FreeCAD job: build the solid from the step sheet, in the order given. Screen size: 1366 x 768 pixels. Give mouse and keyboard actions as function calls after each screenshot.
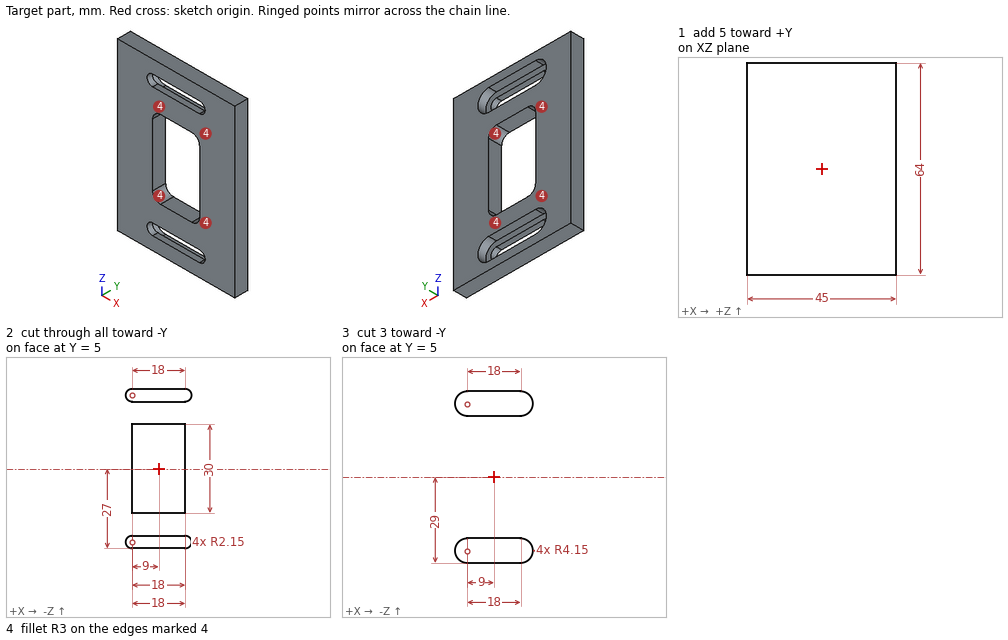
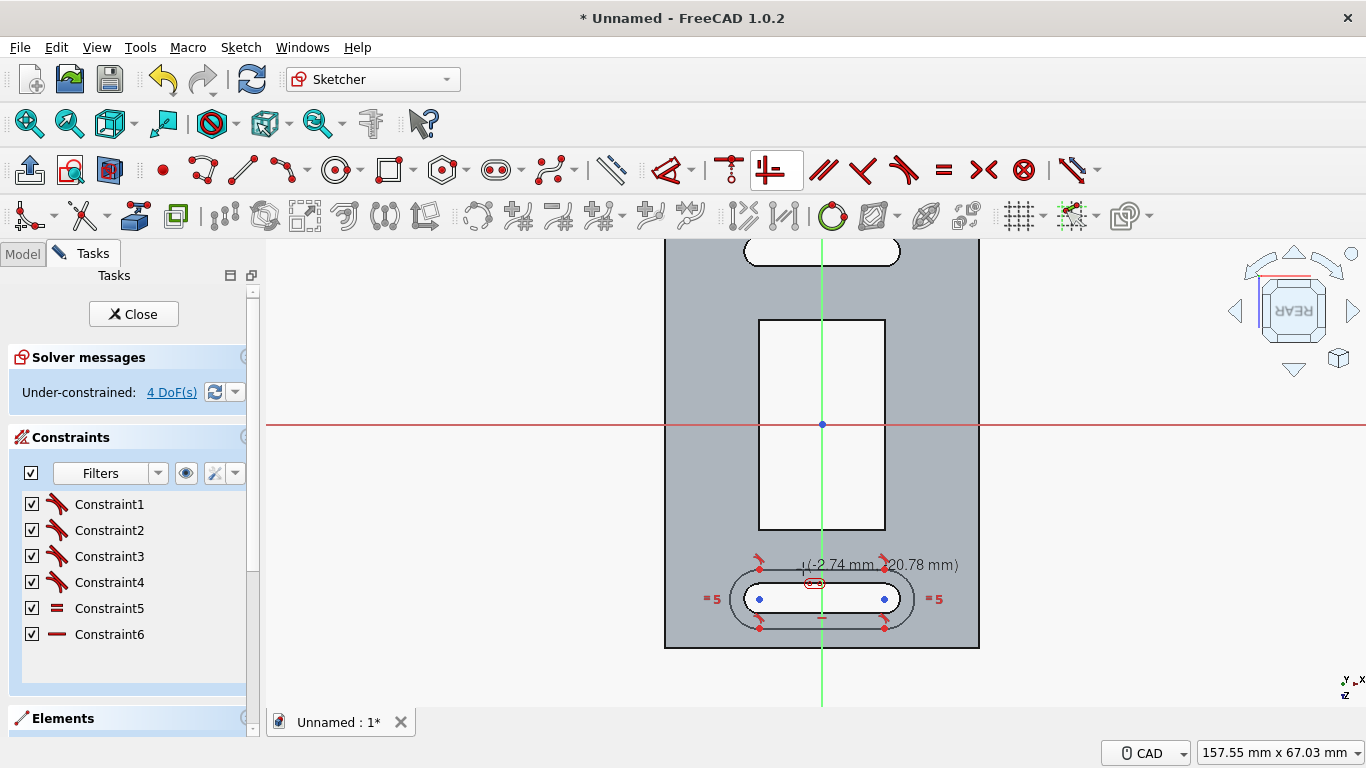
scroll(596, 571, down, 2)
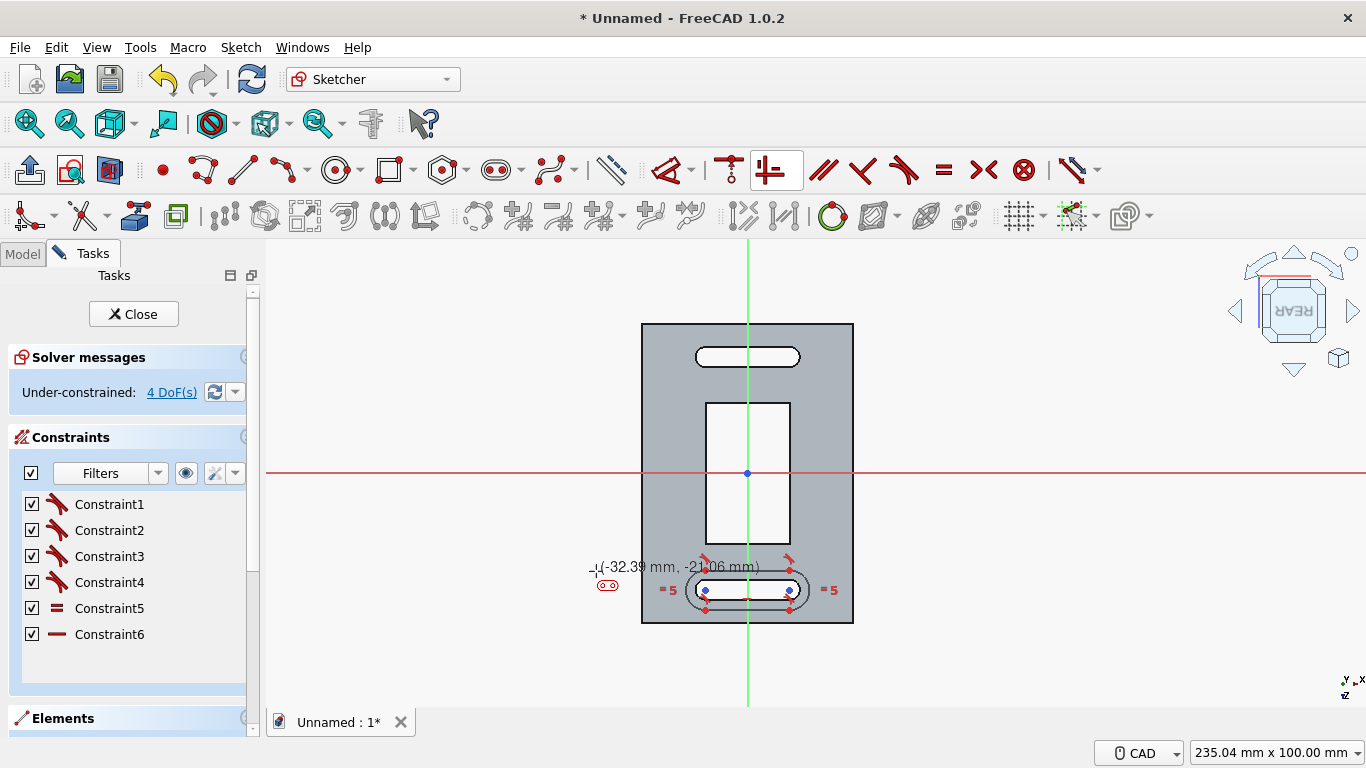
click(706, 357)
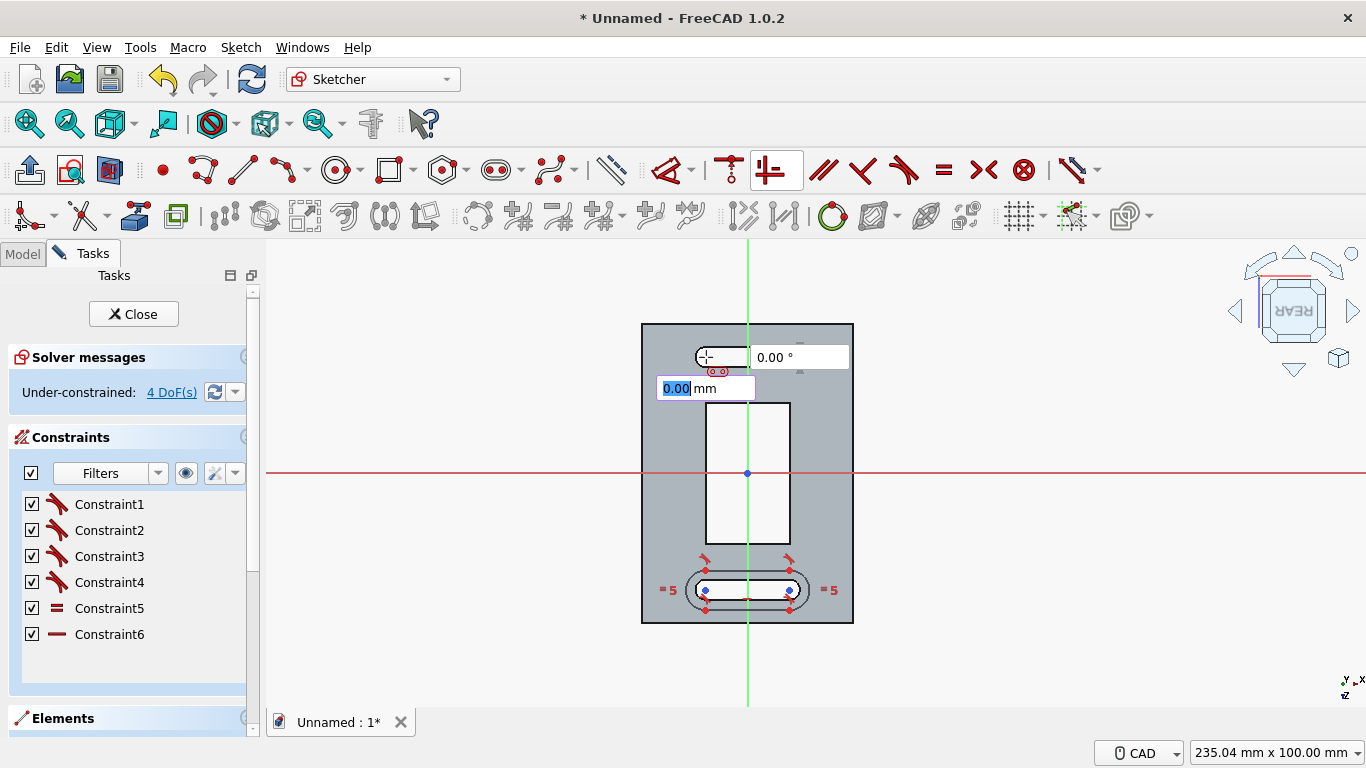
click(790, 357)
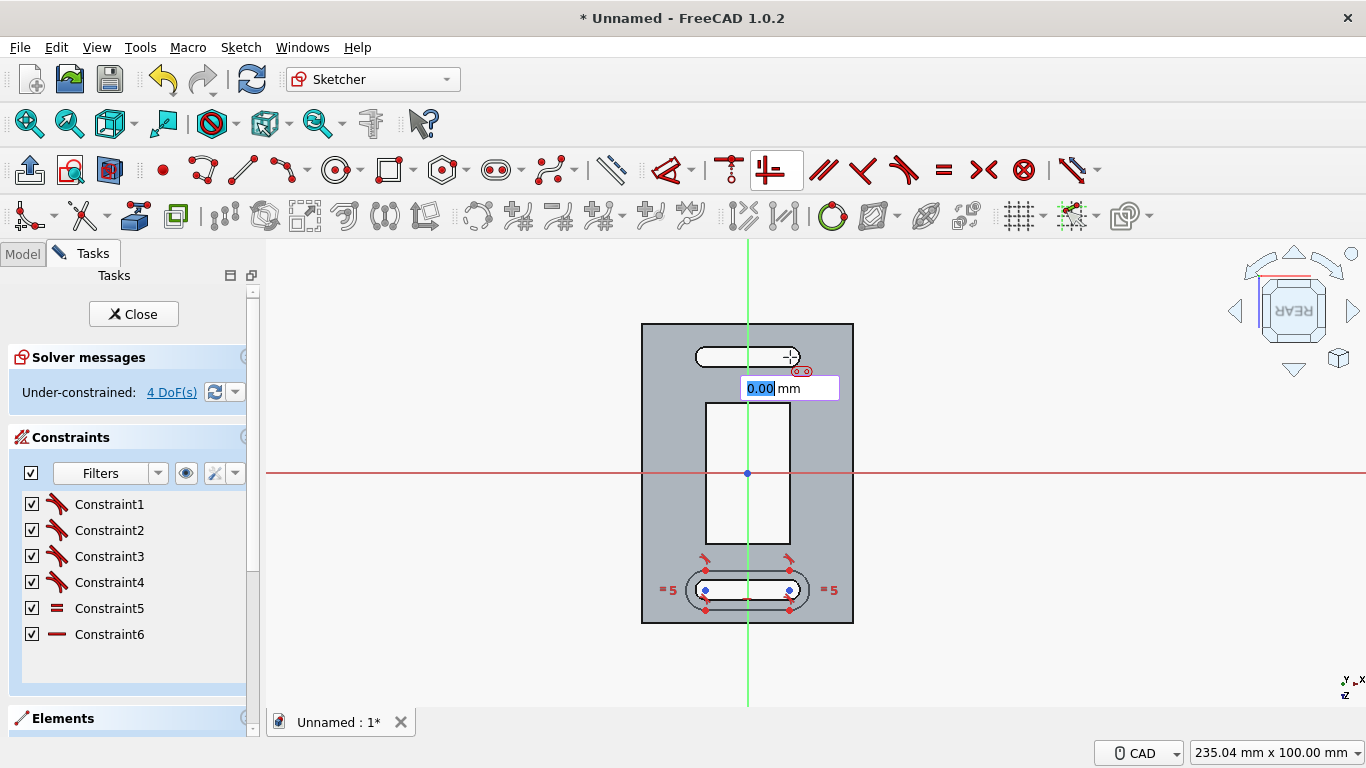
scroll(760, 376, up, 2)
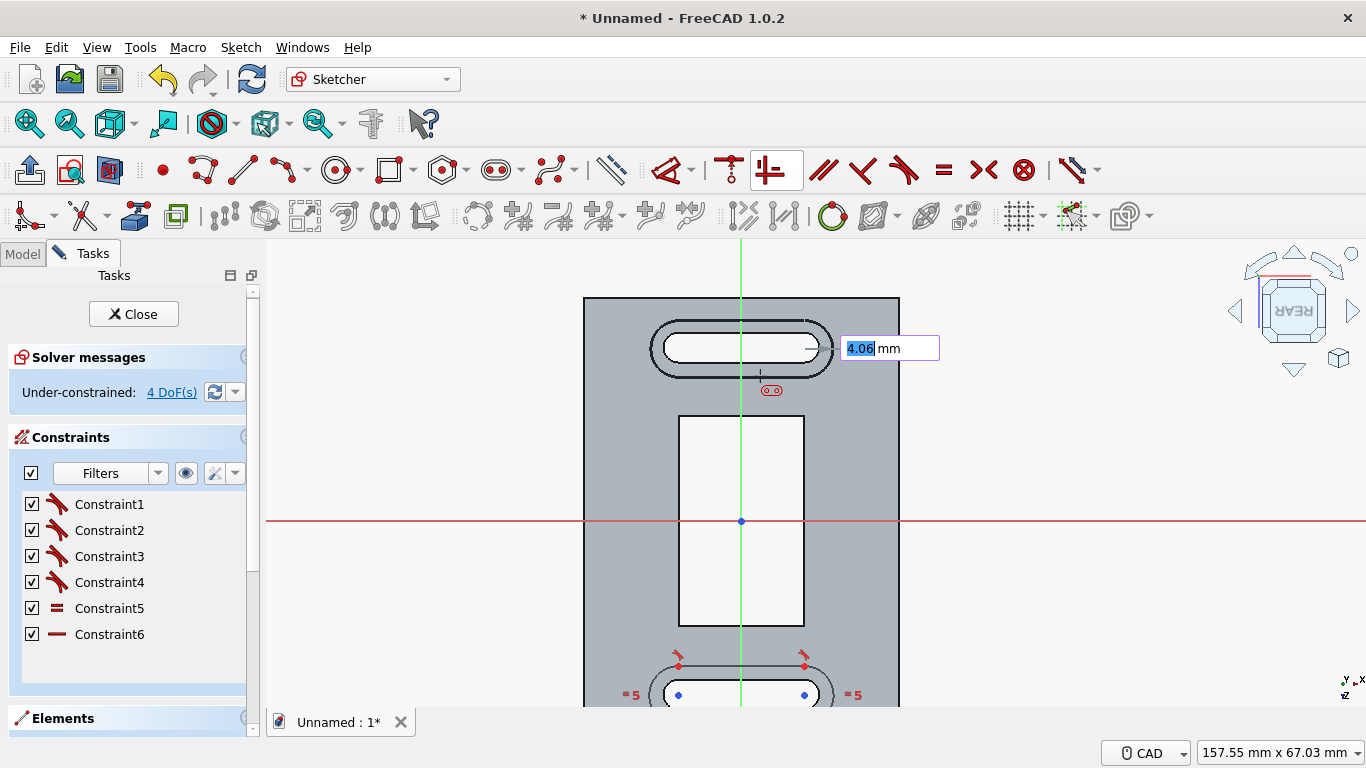
click(760, 377)
key(Escape)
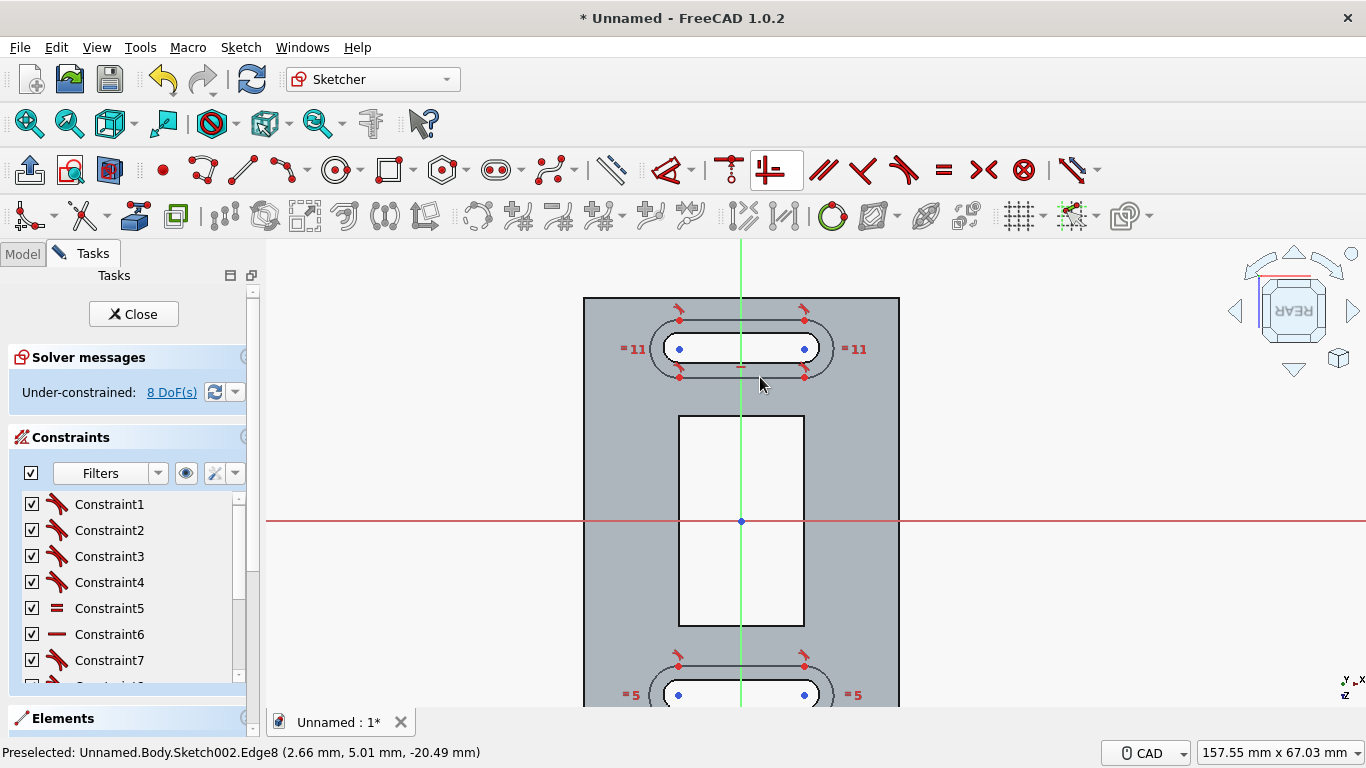
click(655, 678)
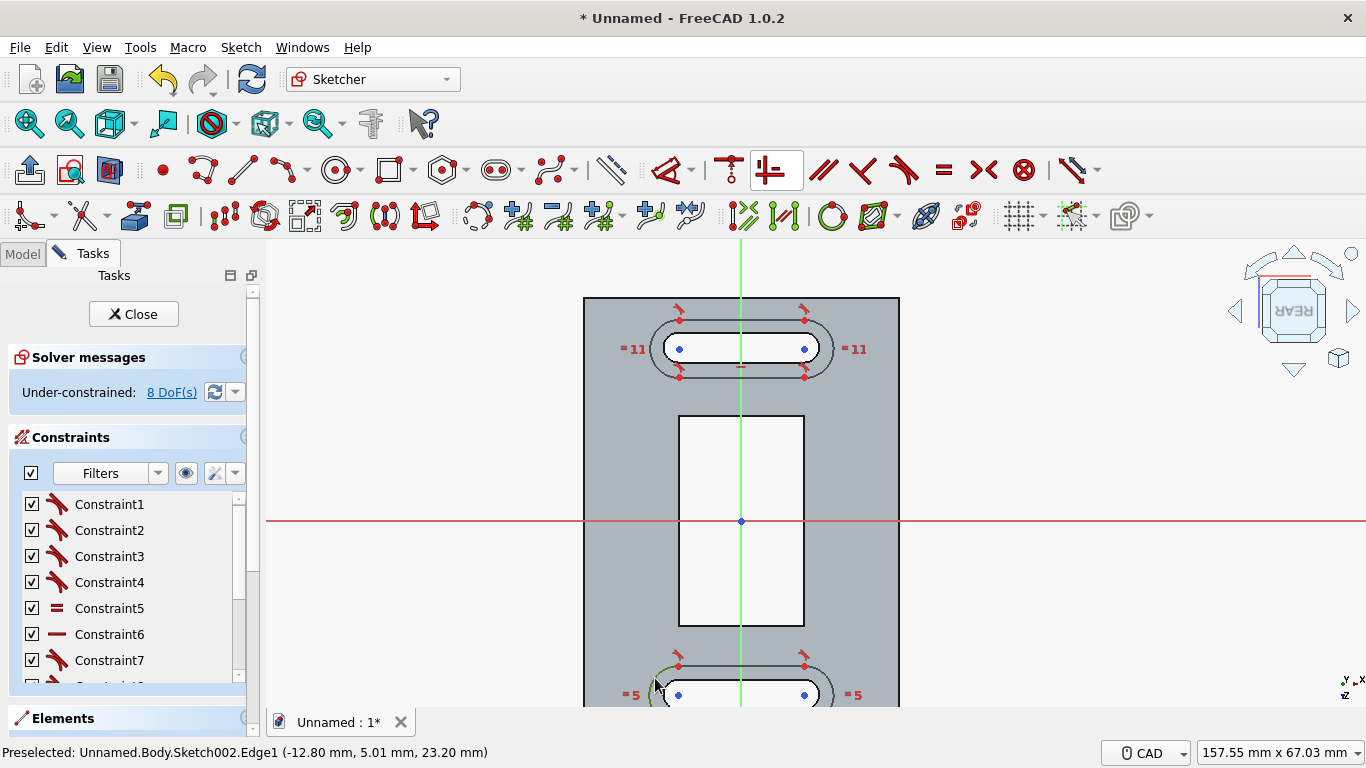
click(656, 332)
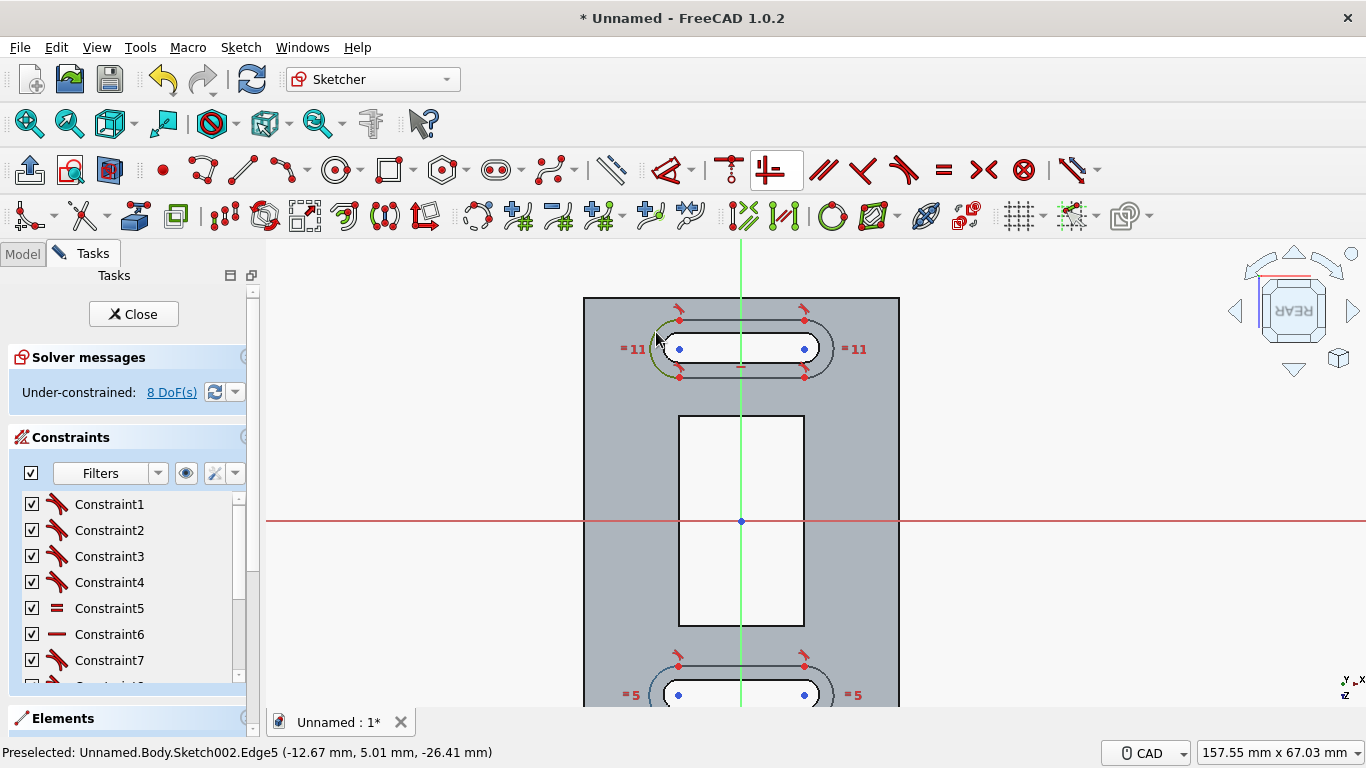
click(944, 170)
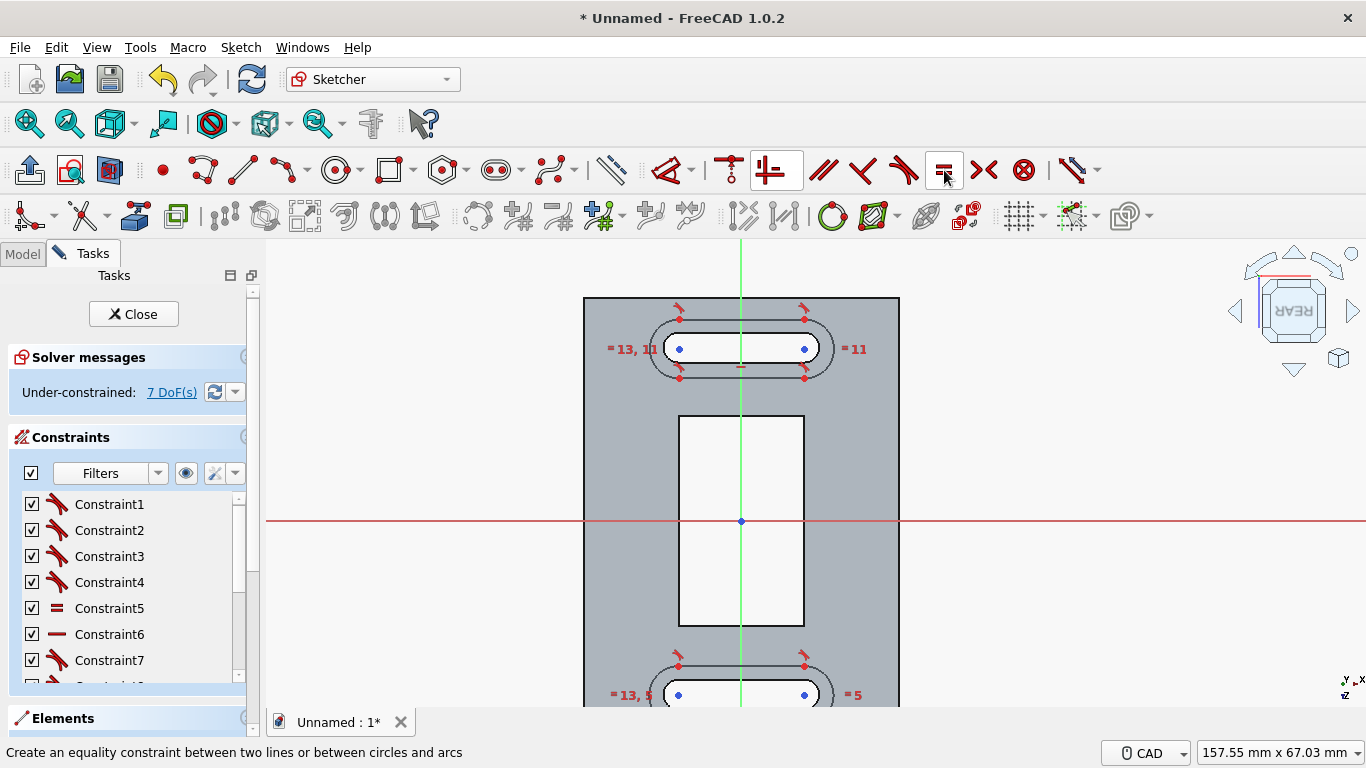
scroll(760, 375, down, 2)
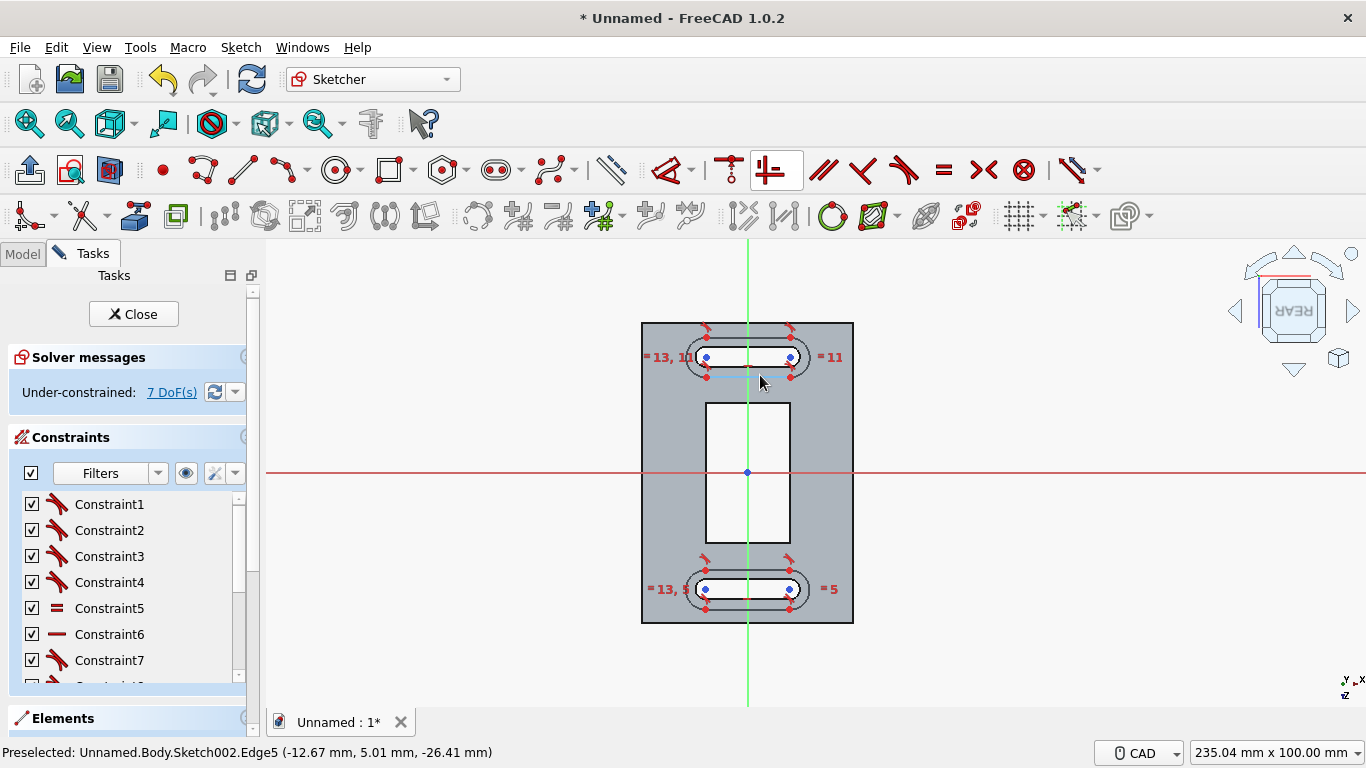
click(706, 590)